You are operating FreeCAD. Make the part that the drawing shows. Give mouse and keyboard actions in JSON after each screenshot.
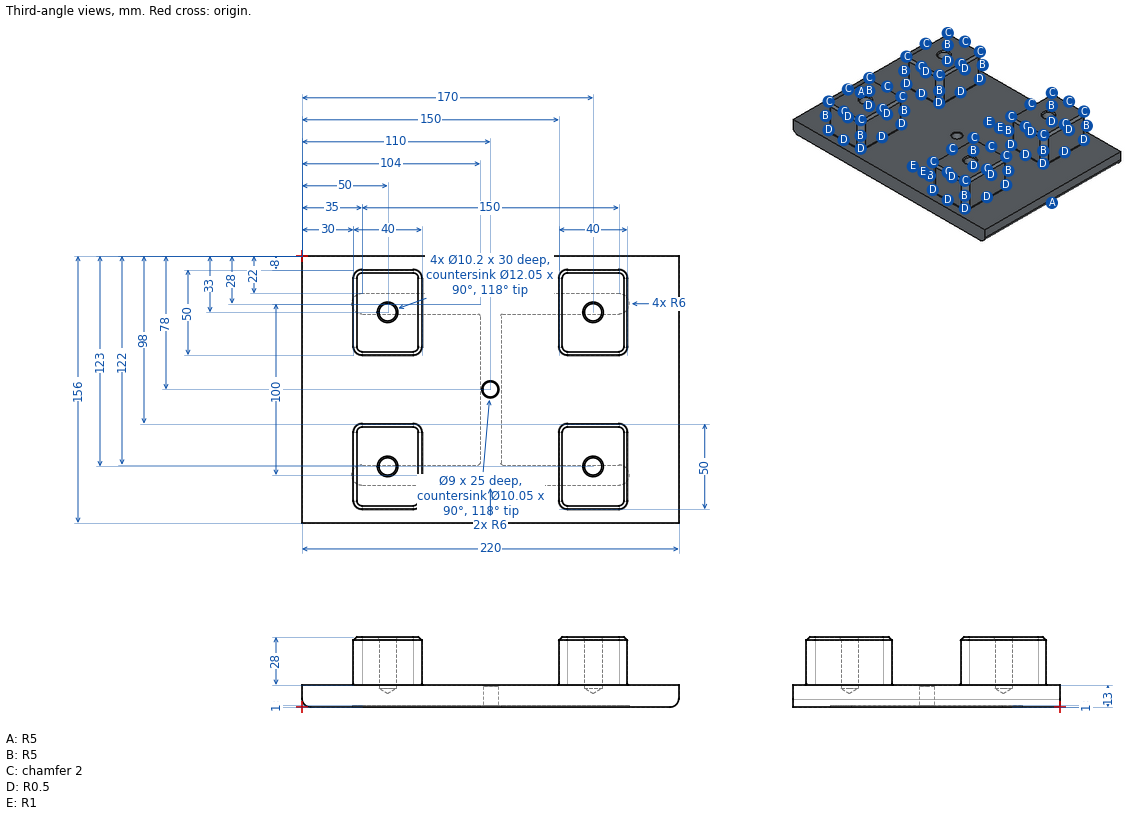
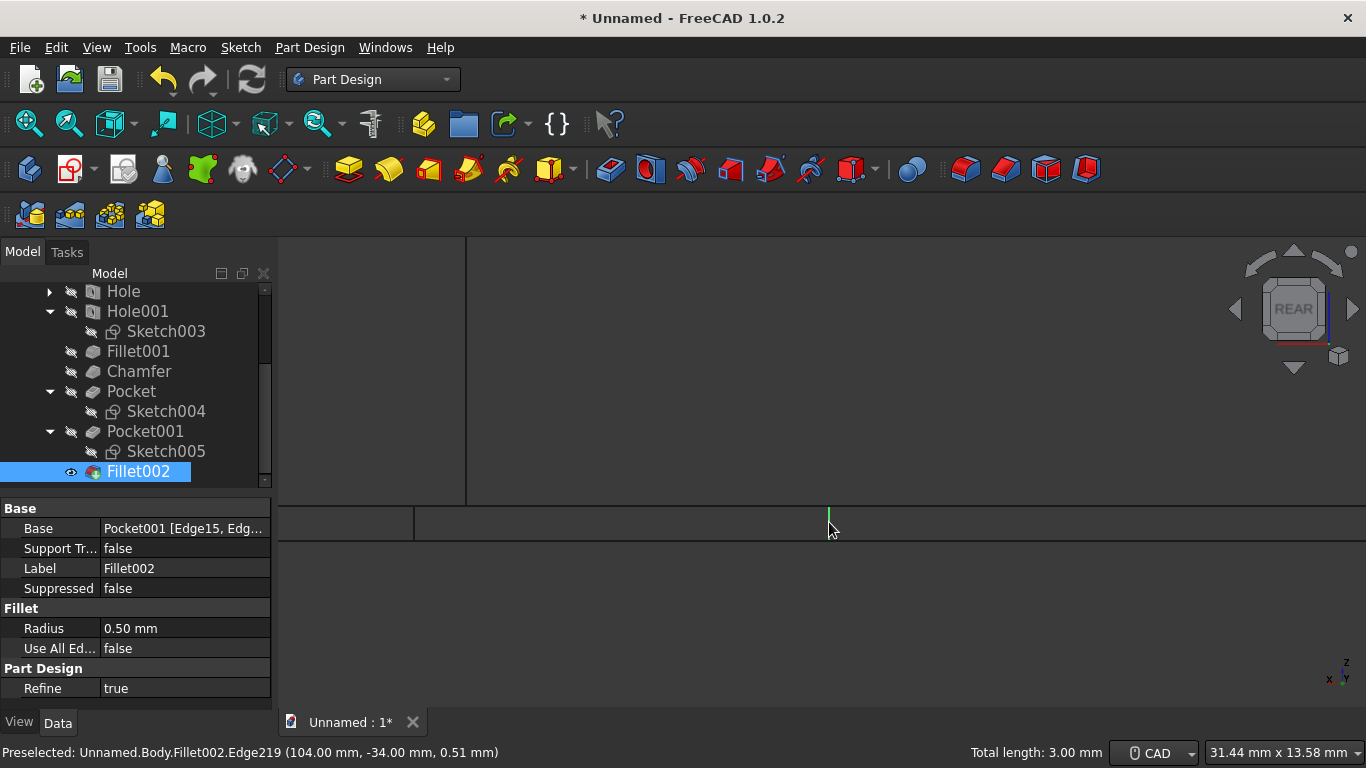
{"action": "left_click", "coordinate": [414, 522], "text": "ctrl"}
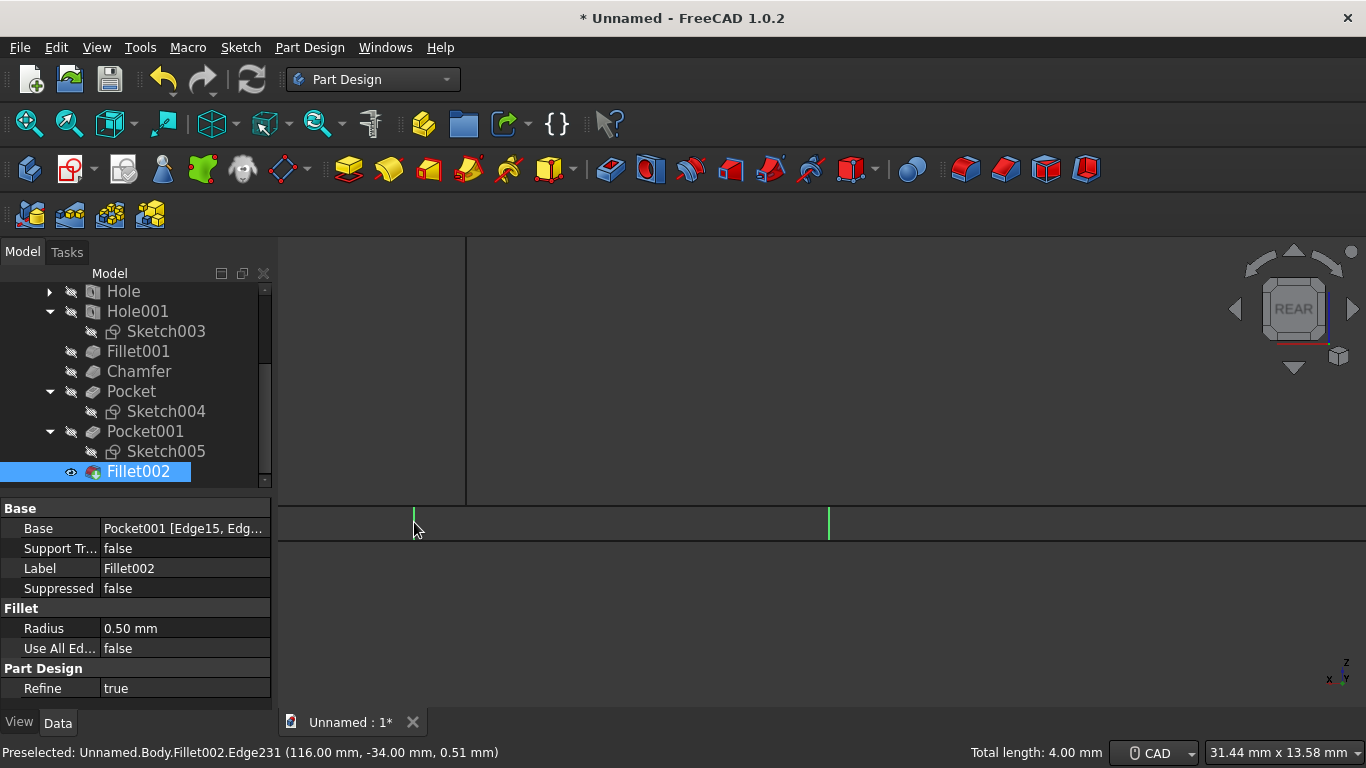
{"action": "key", "text": "v 1"}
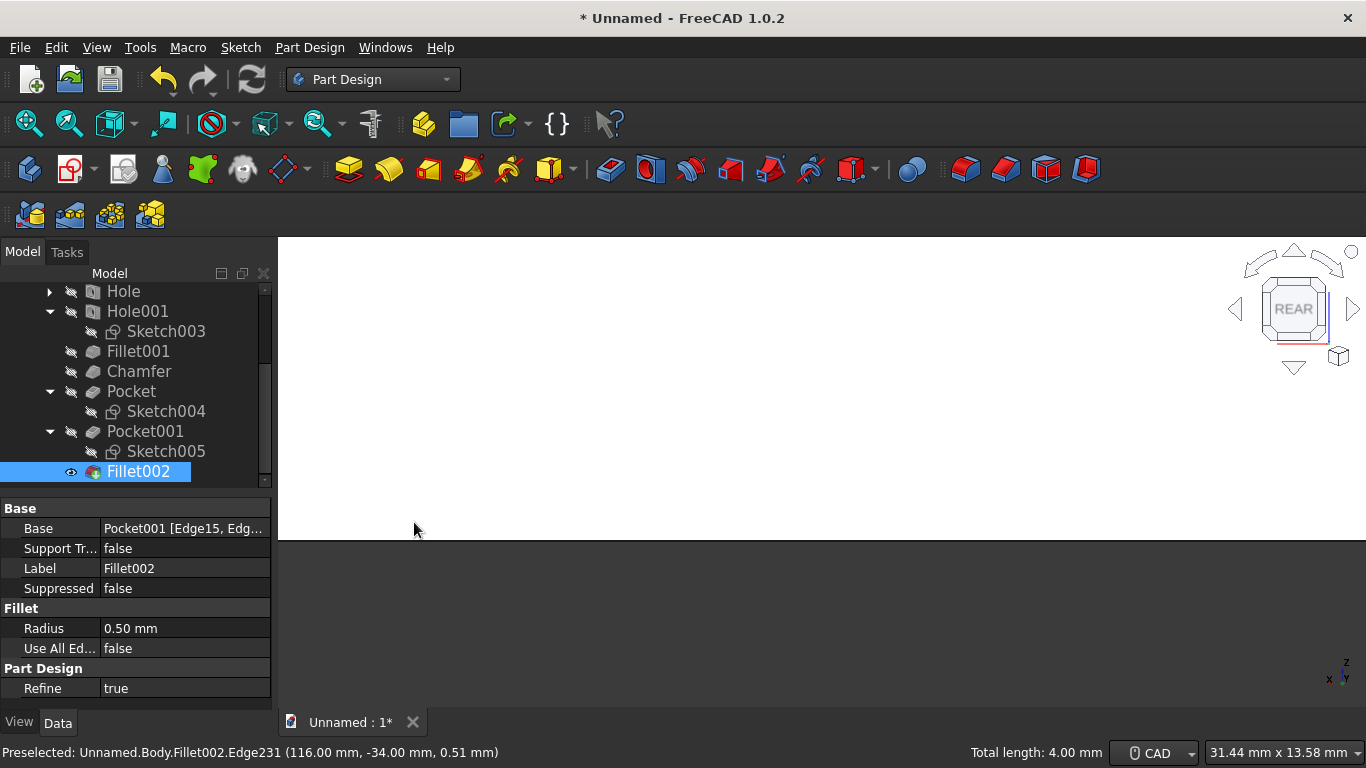
{"action": "left_click", "coordinate": [966, 170]}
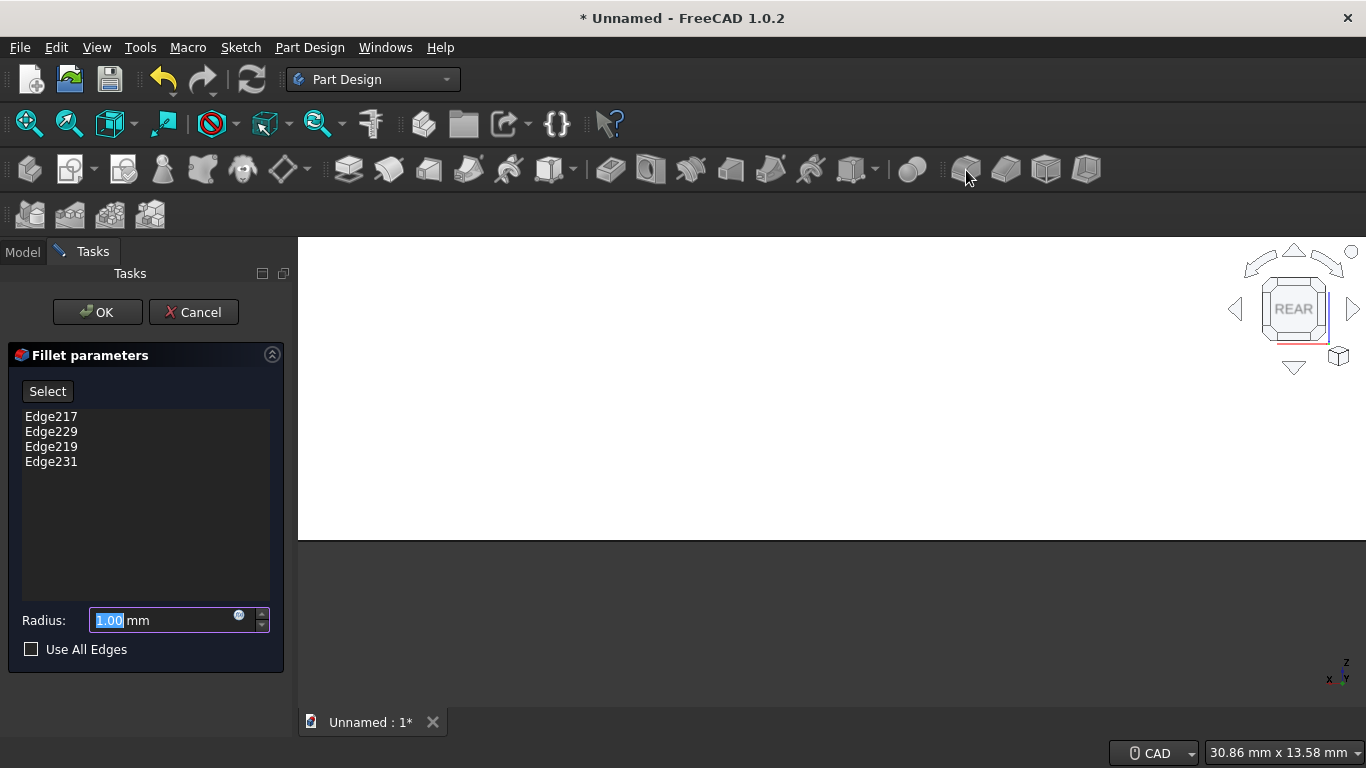
{"action": "type", "text": "1"}
{"action": "key", "text": "Tab"}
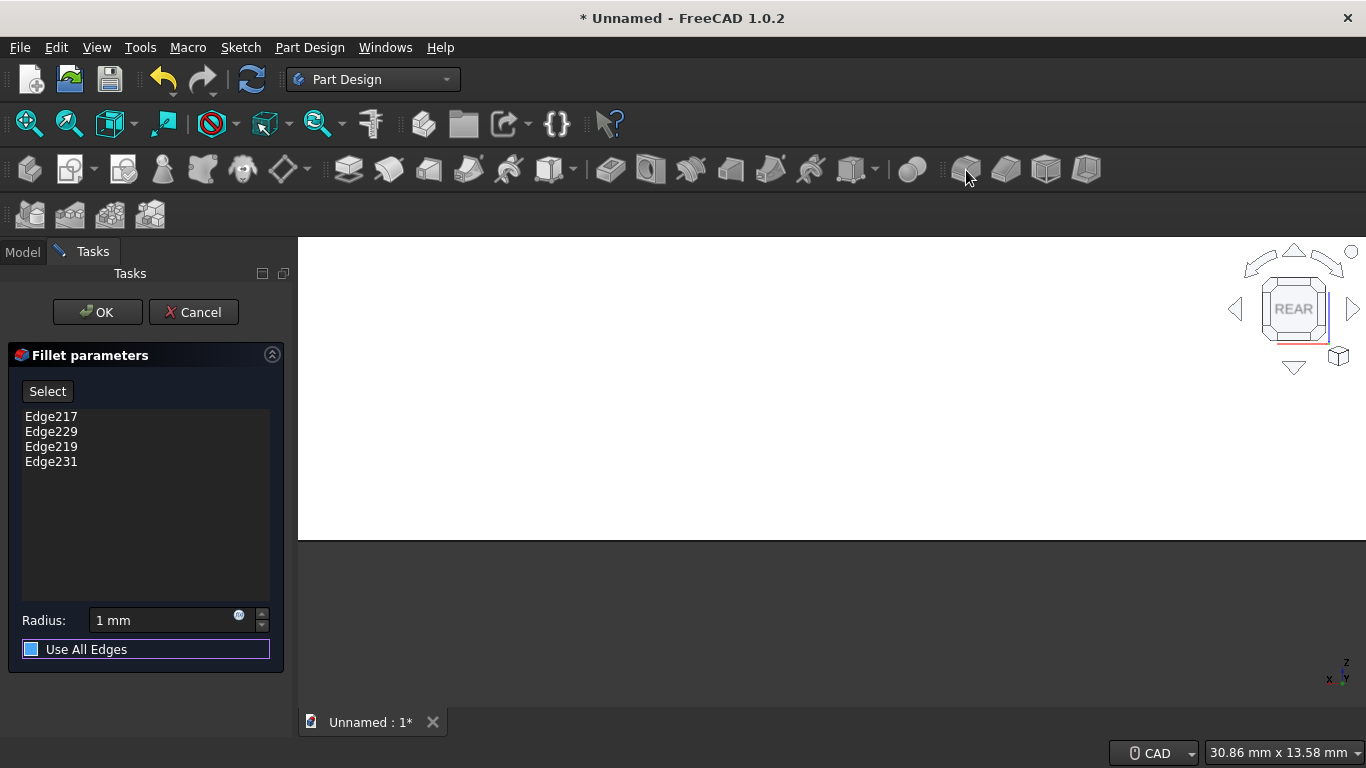
{"action": "left_click", "coordinate": [98, 312]}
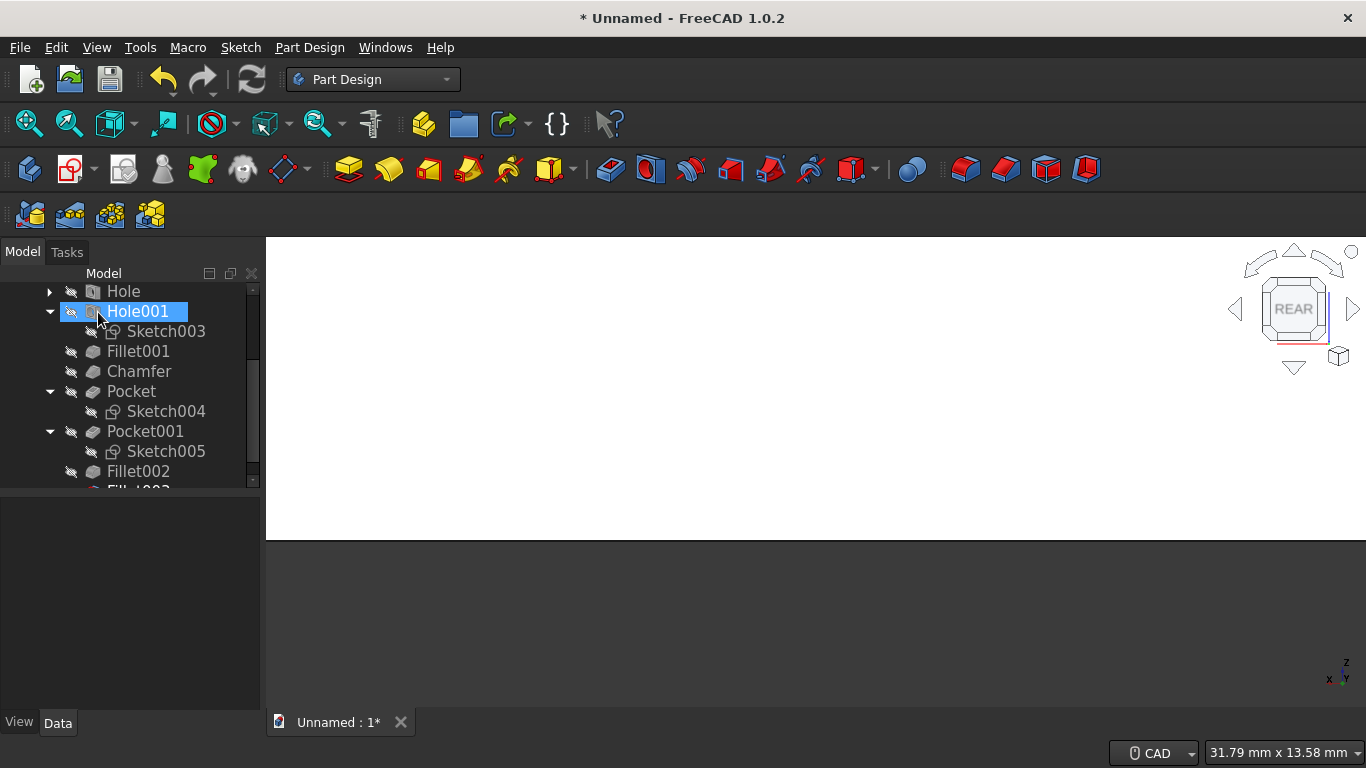
{"action": "key", "text": "0"}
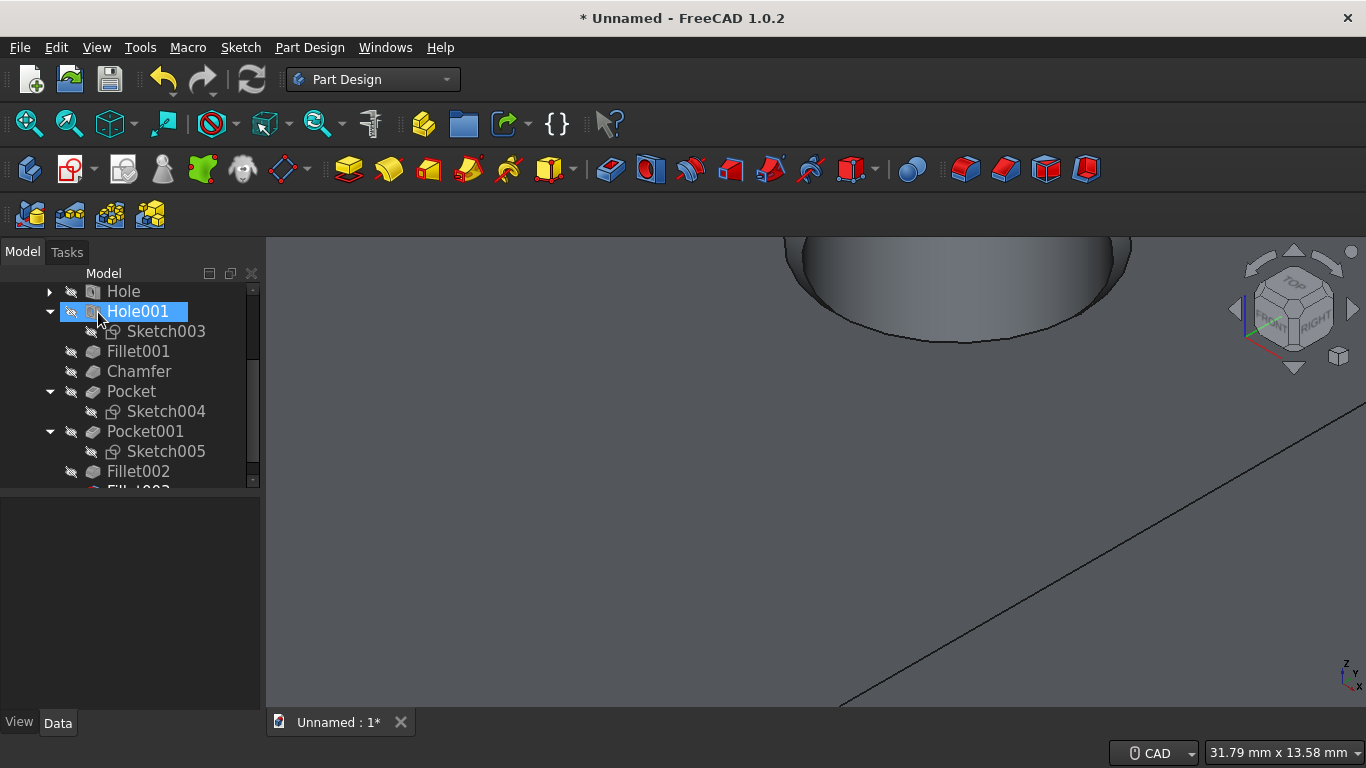
{"action": "key", "text": "v f"}